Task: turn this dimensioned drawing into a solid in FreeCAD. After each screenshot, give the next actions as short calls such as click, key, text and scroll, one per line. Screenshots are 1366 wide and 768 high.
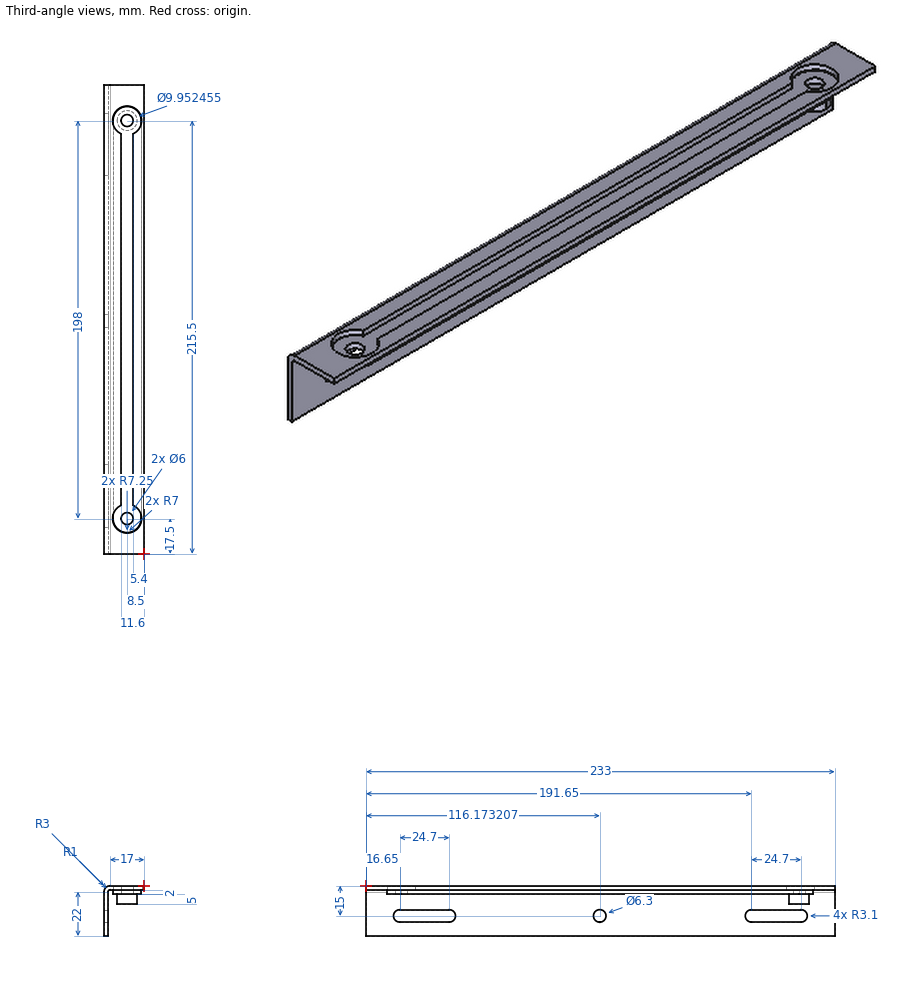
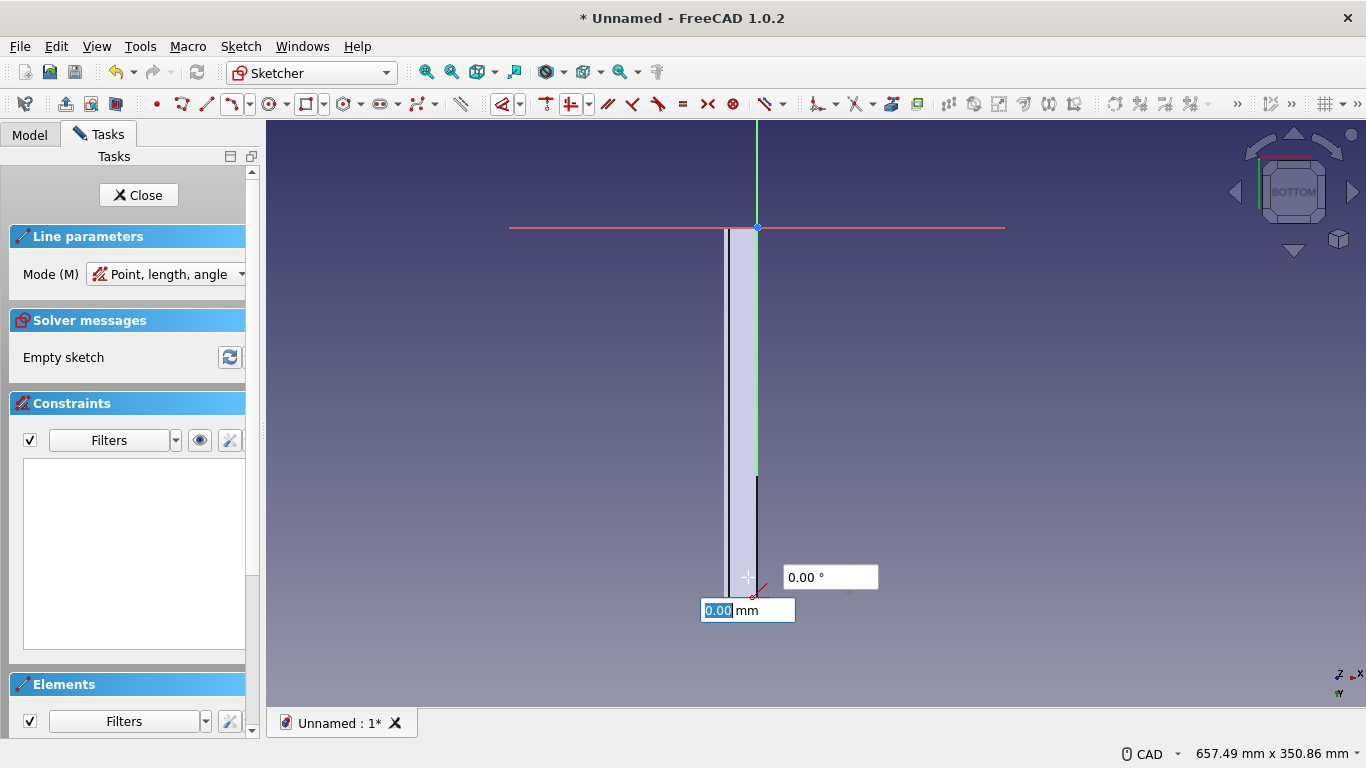
scroll(748, 268, up, 3)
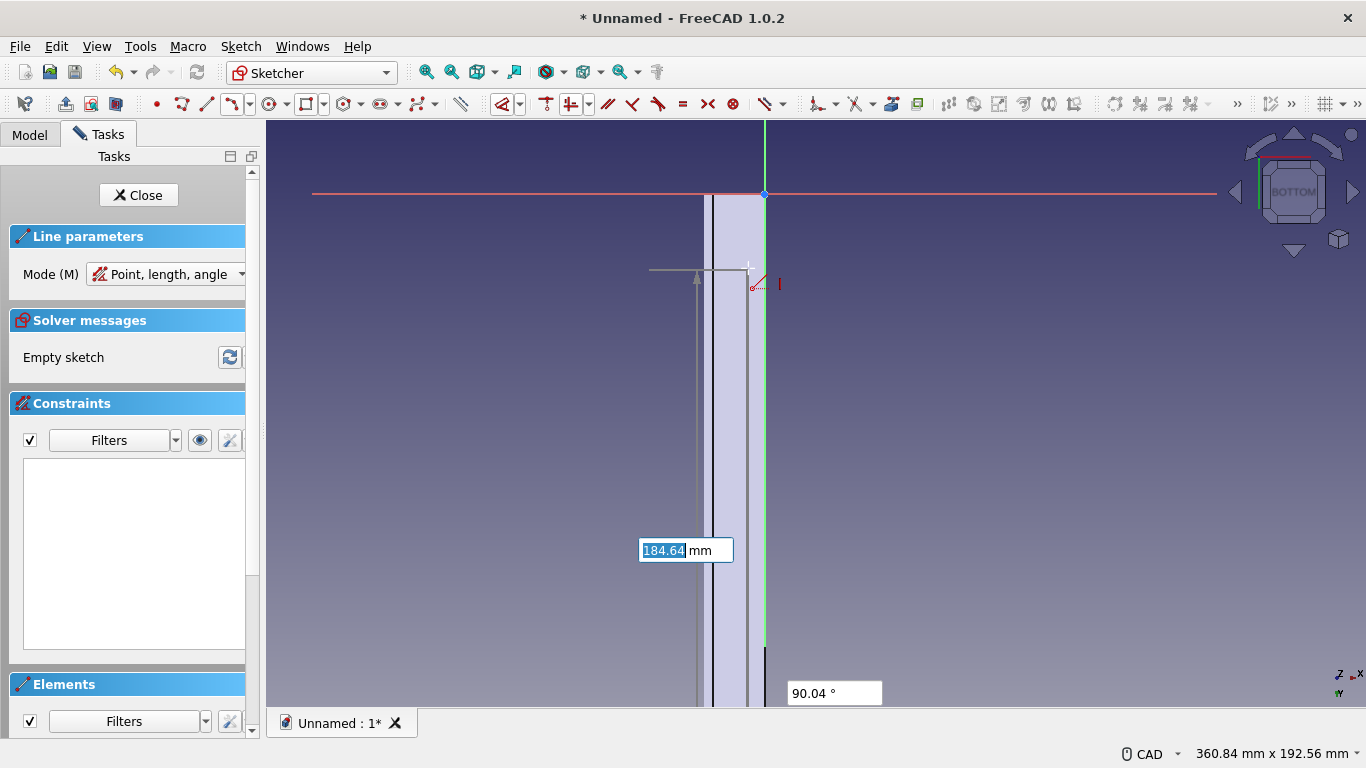
click(748, 267)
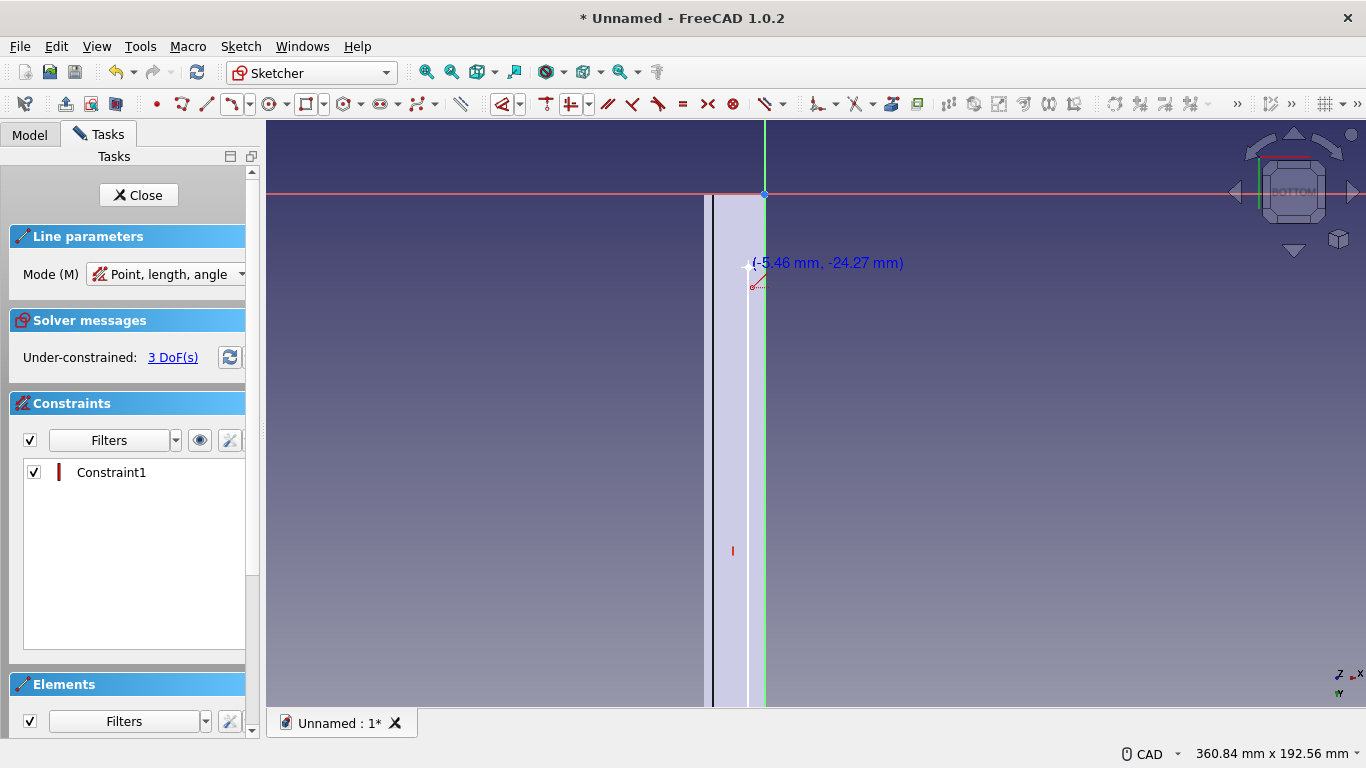
click(729, 267)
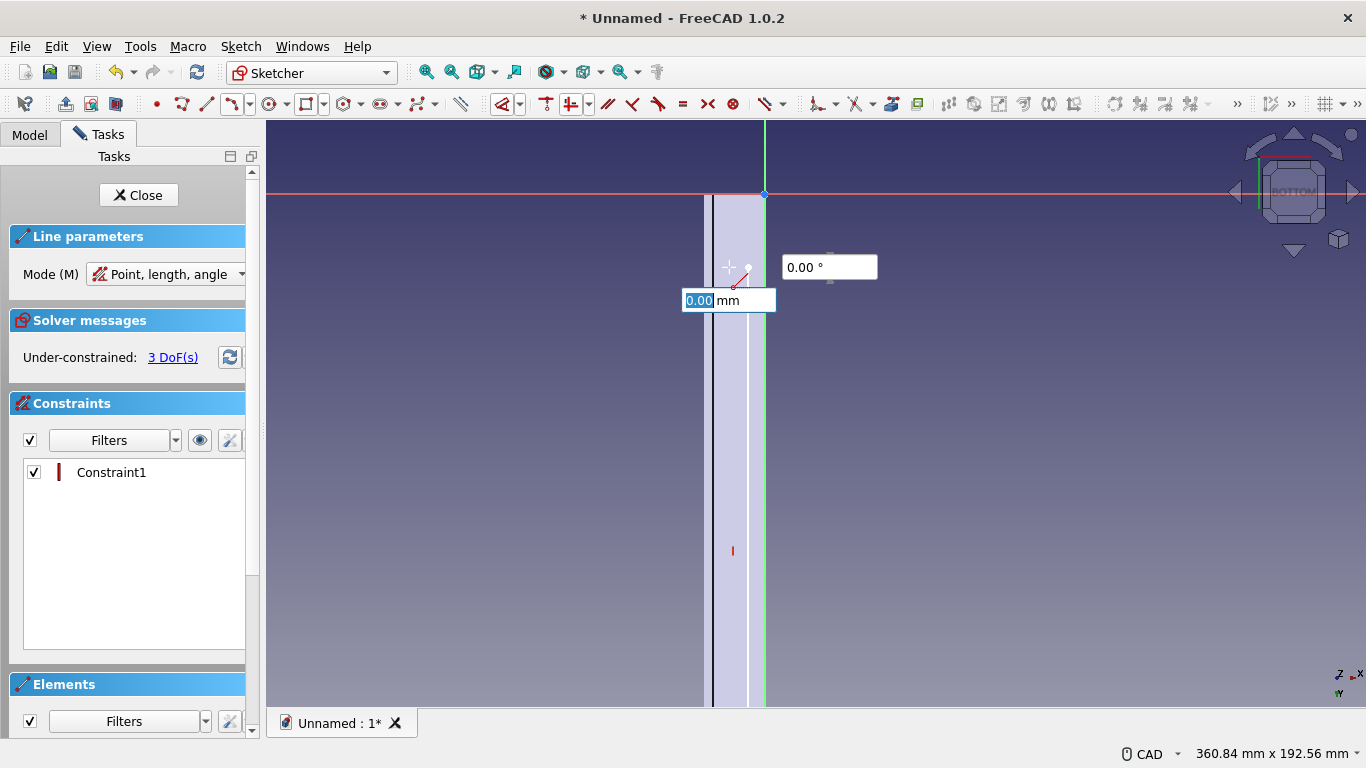
scroll(748, 267, down, 3)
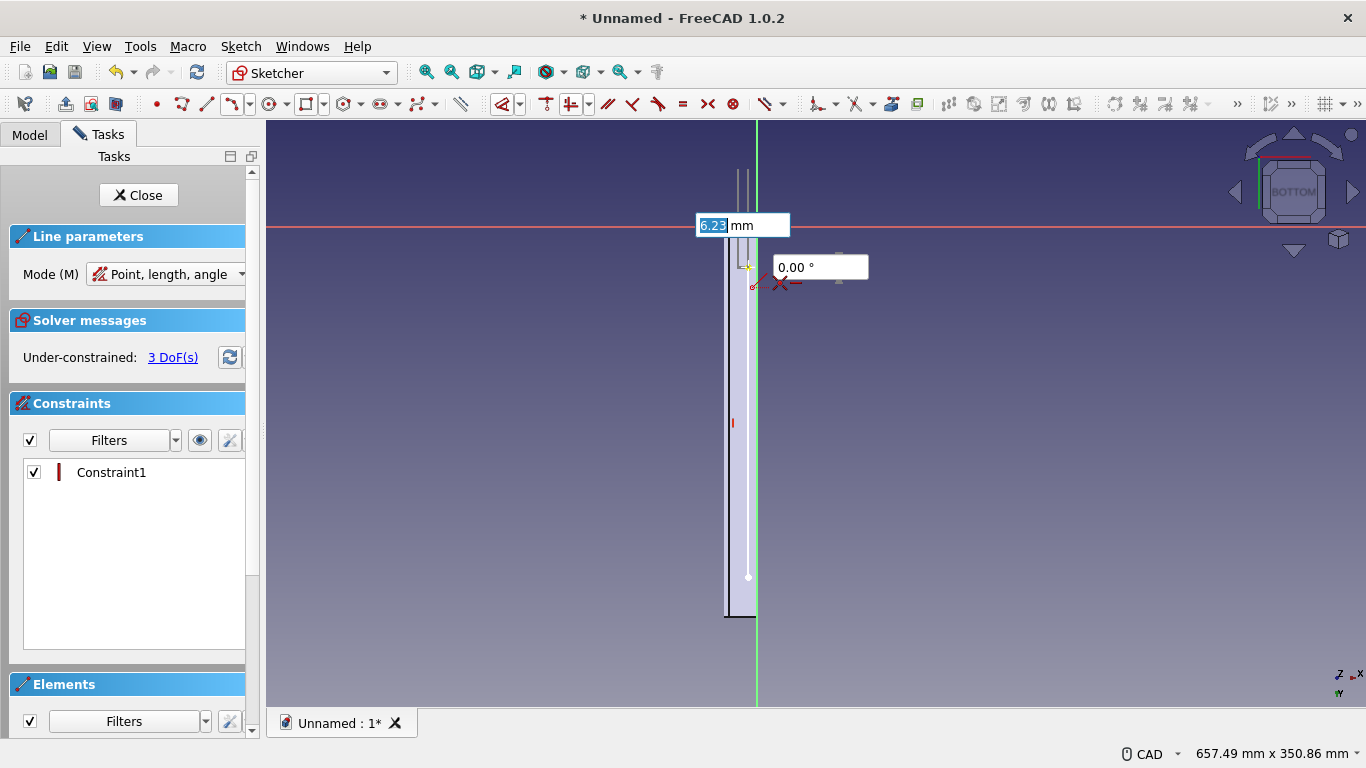
scroll(738, 577, up, 3)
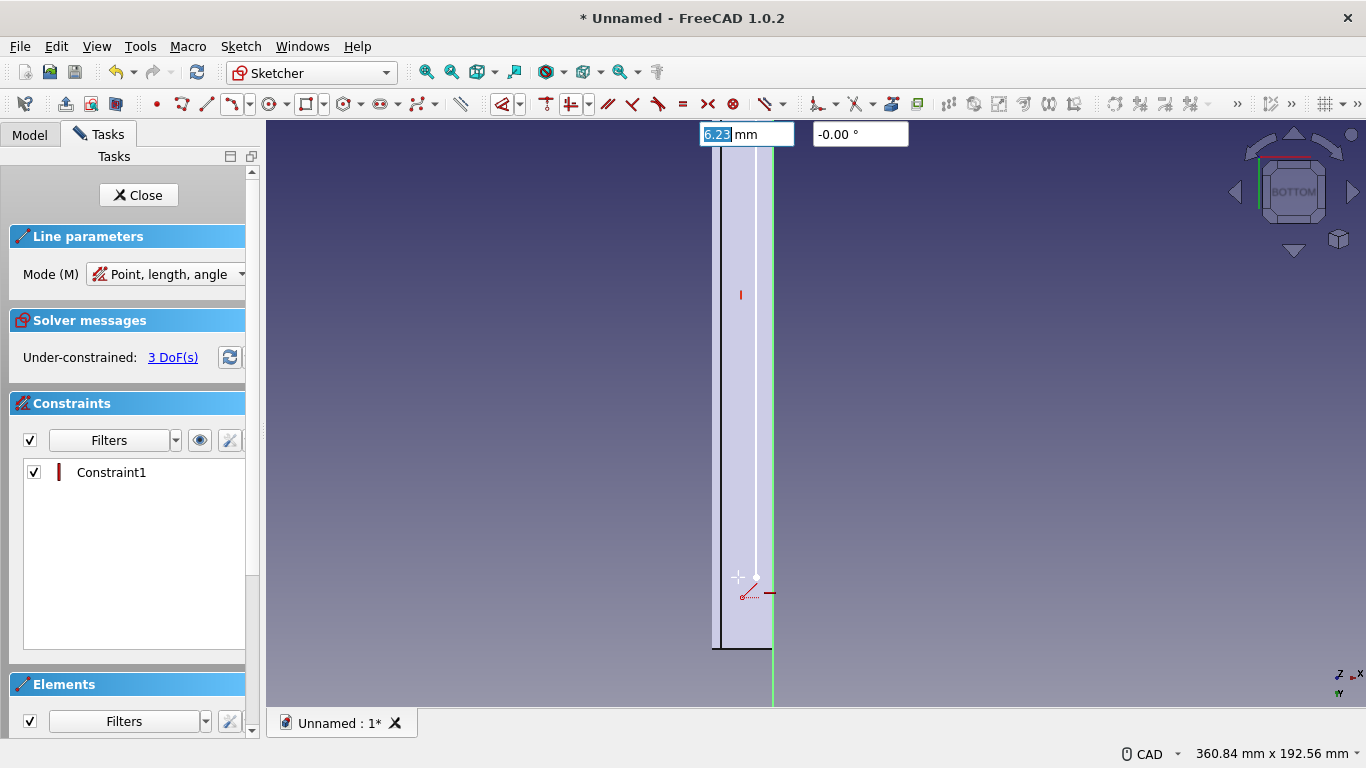
click(737, 576)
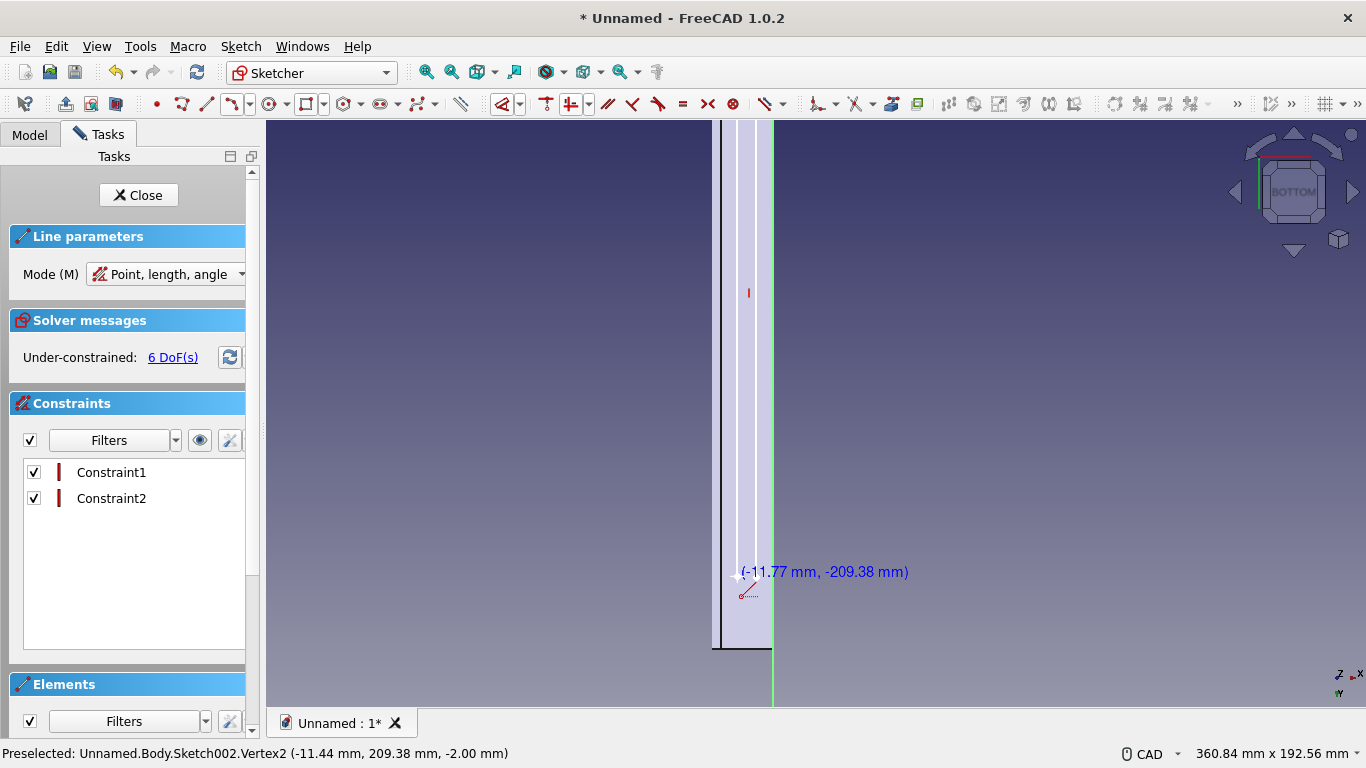
click(232, 104)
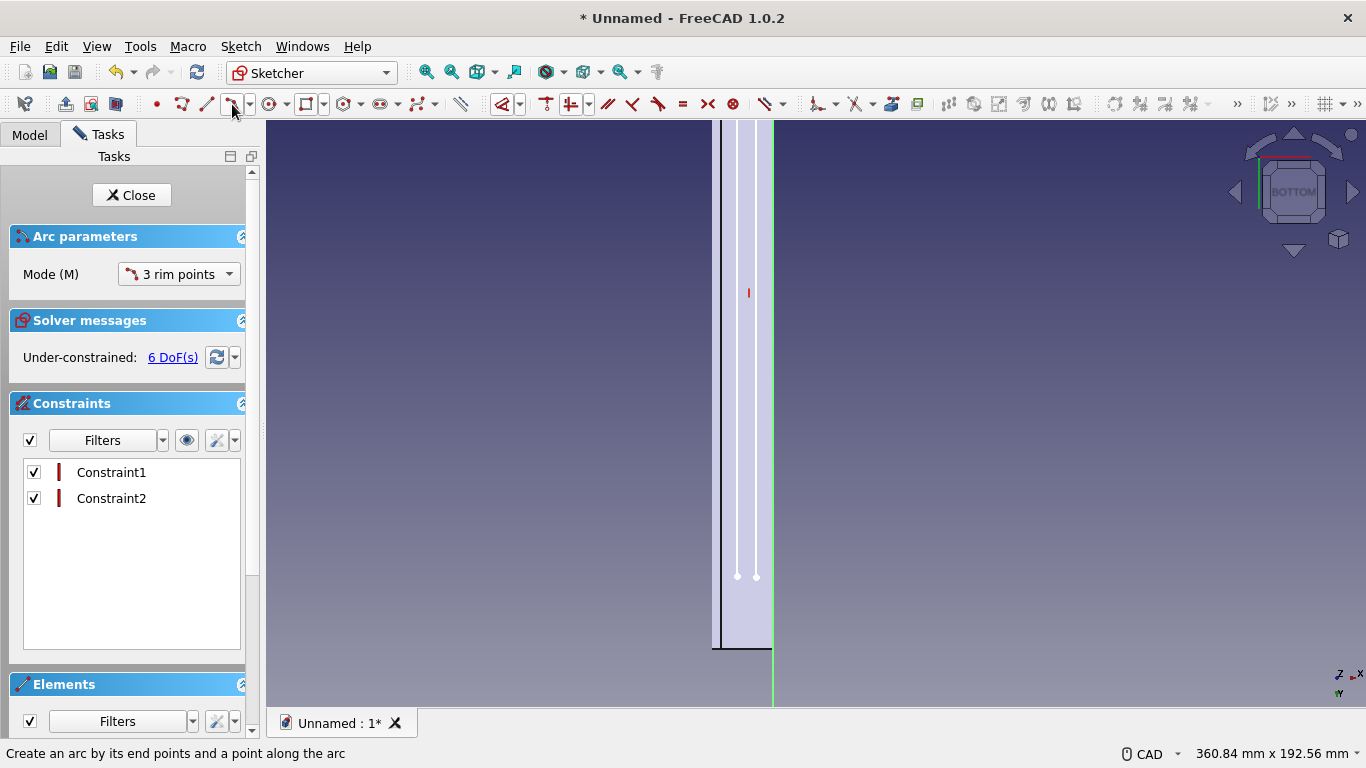
scroll(738, 578, down, 3)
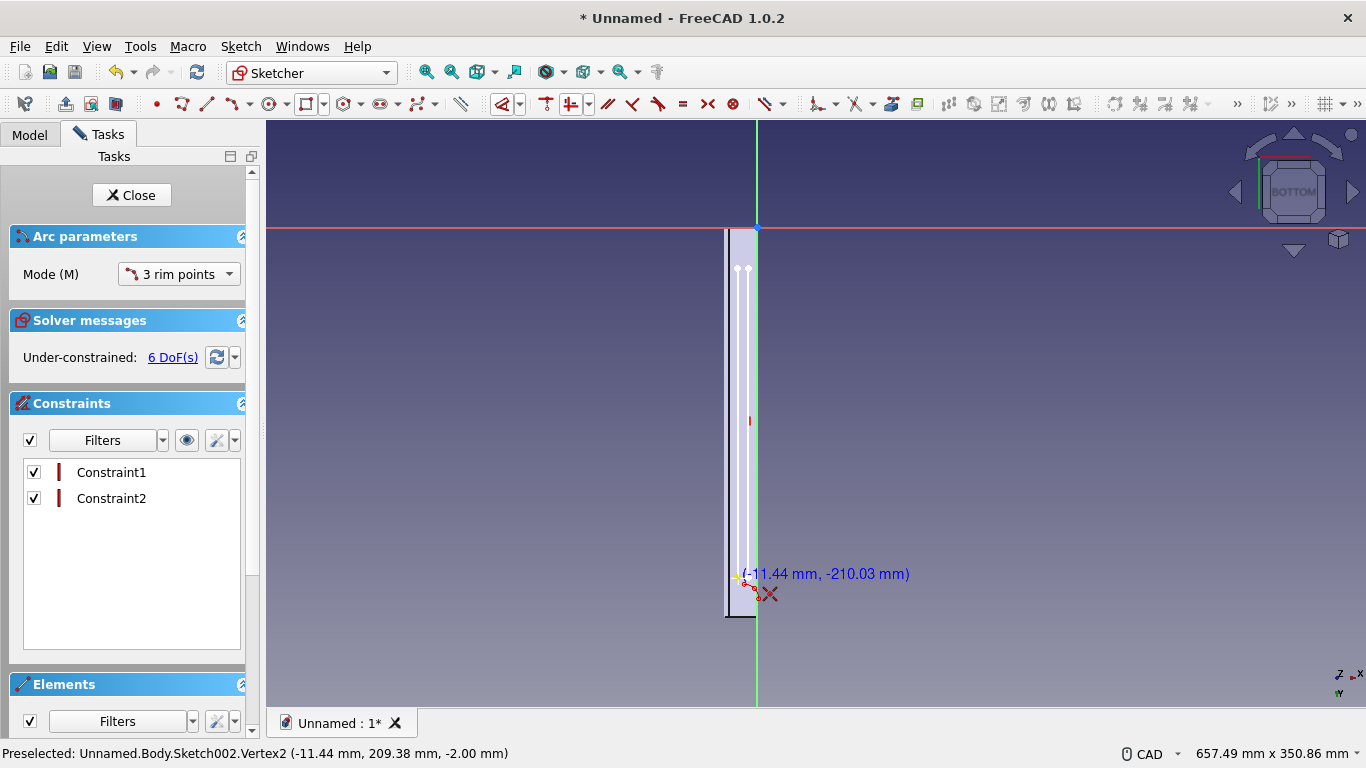
scroll(748, 268, up, 3)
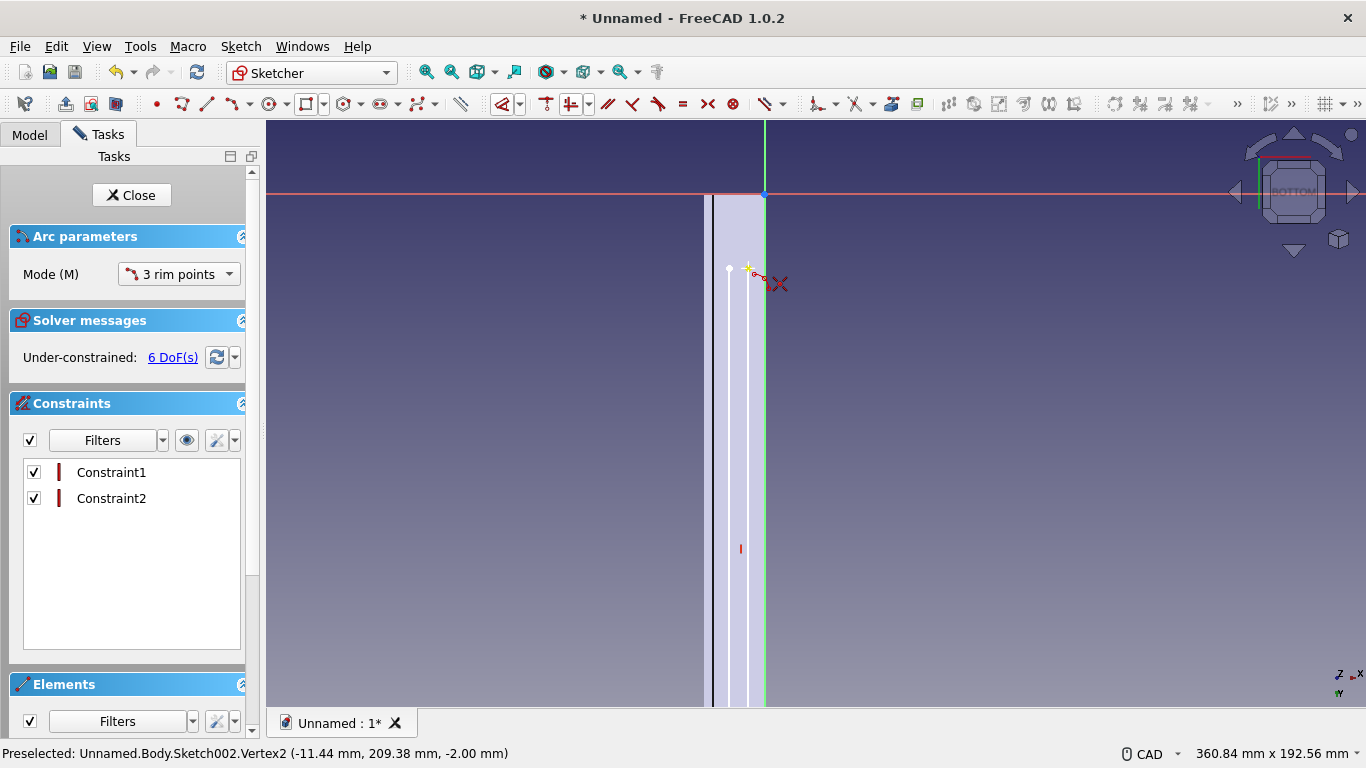
click(748, 268)
click(729, 268)
click(739, 225)